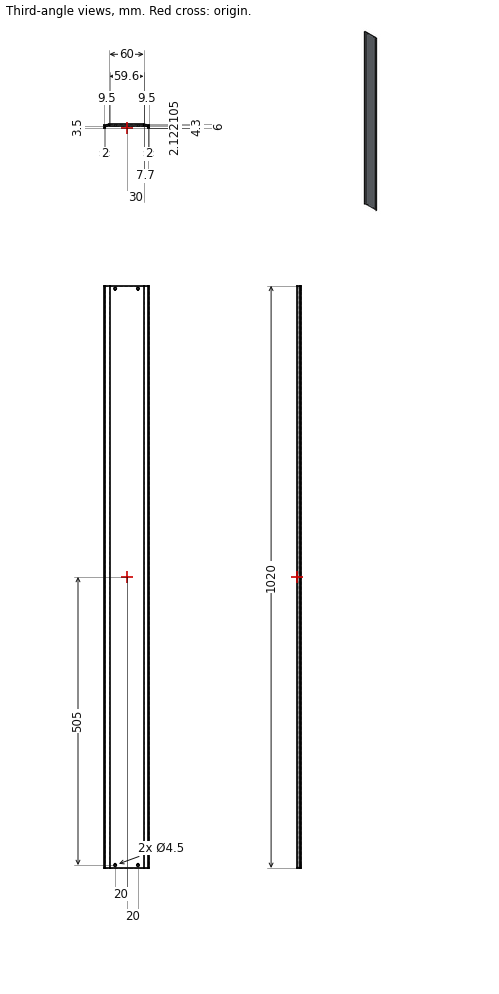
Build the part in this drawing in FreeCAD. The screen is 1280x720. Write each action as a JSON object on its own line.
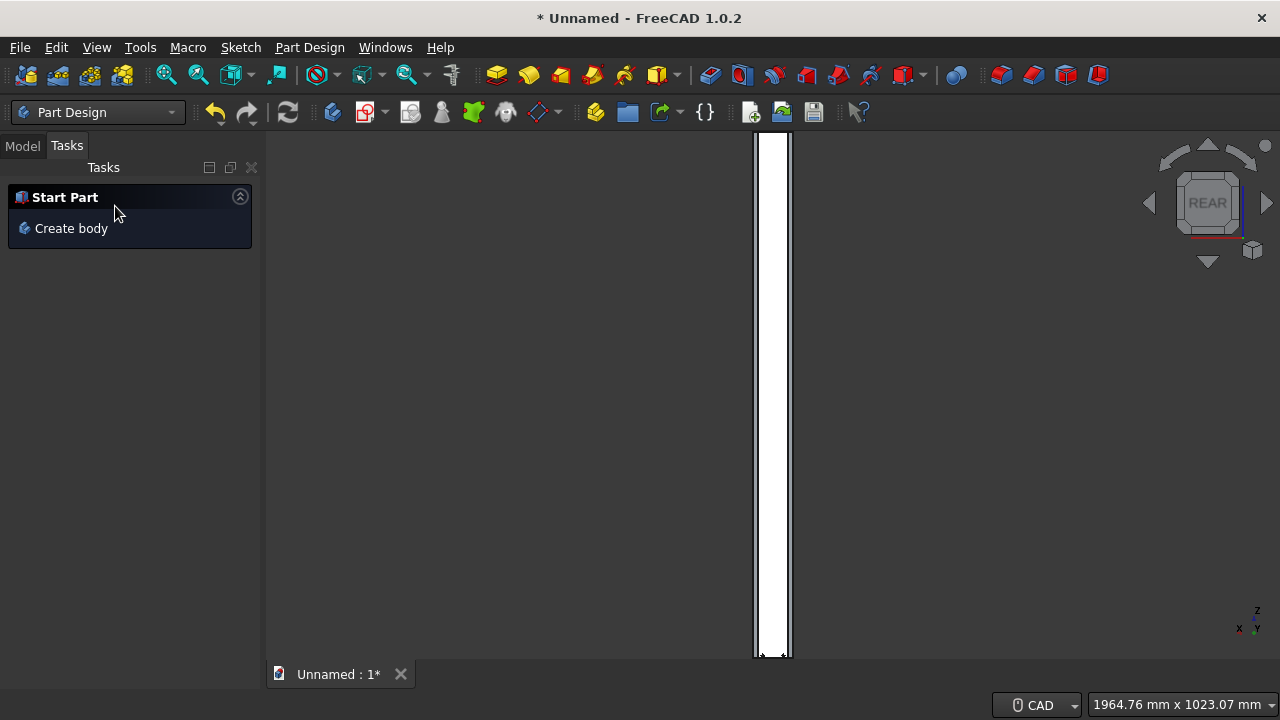
{"action": "left_click", "coordinate": [23, 145]}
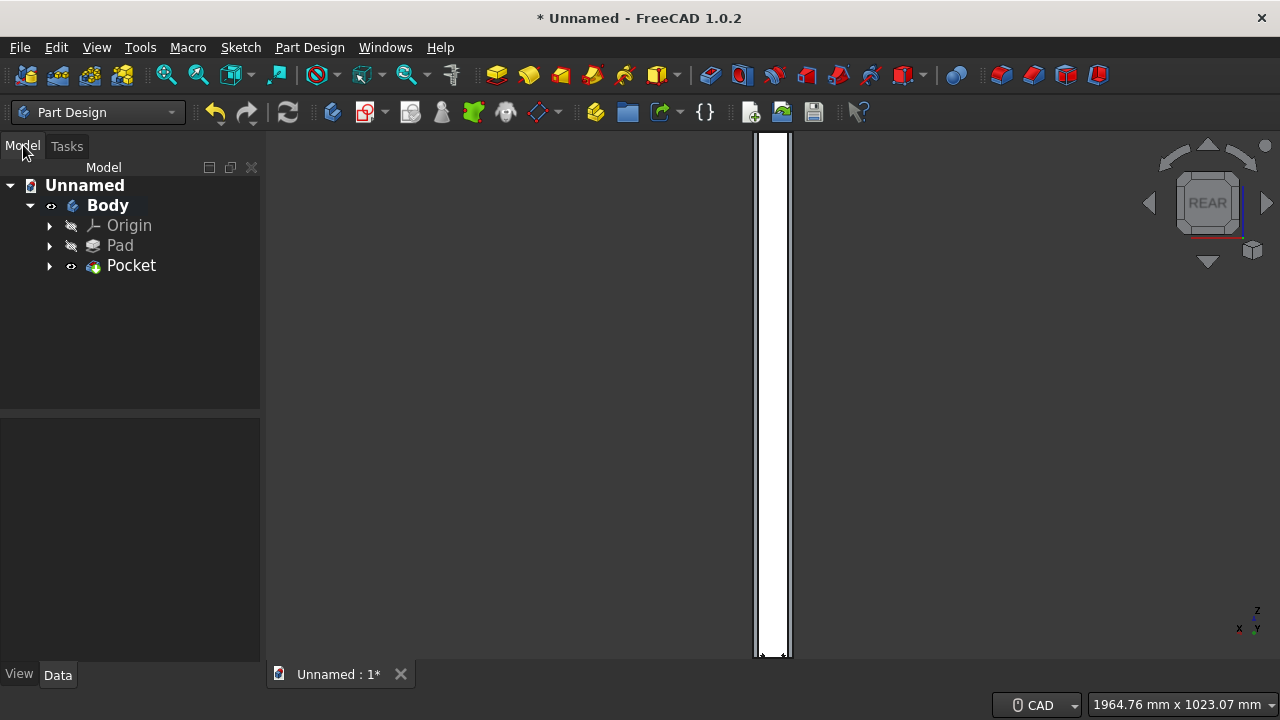
{"action": "left_click", "coordinate": [116, 266]}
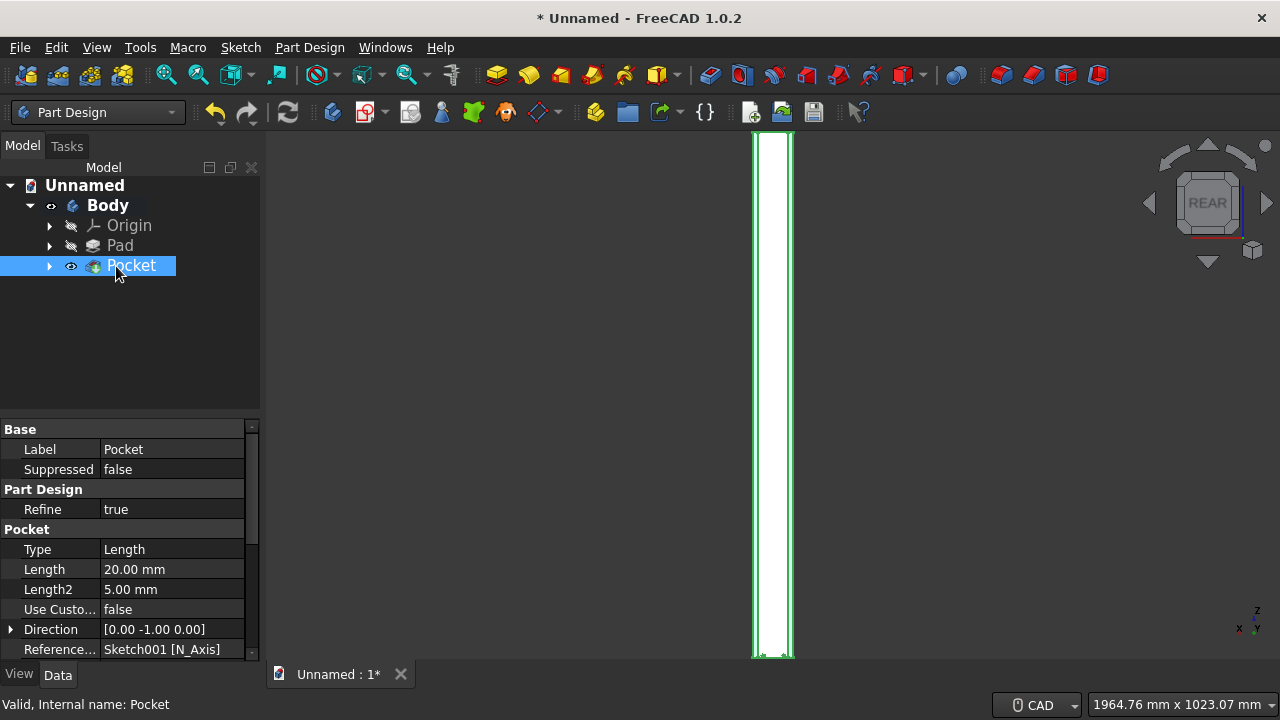
{"action": "left_click", "coordinate": [26, 76]}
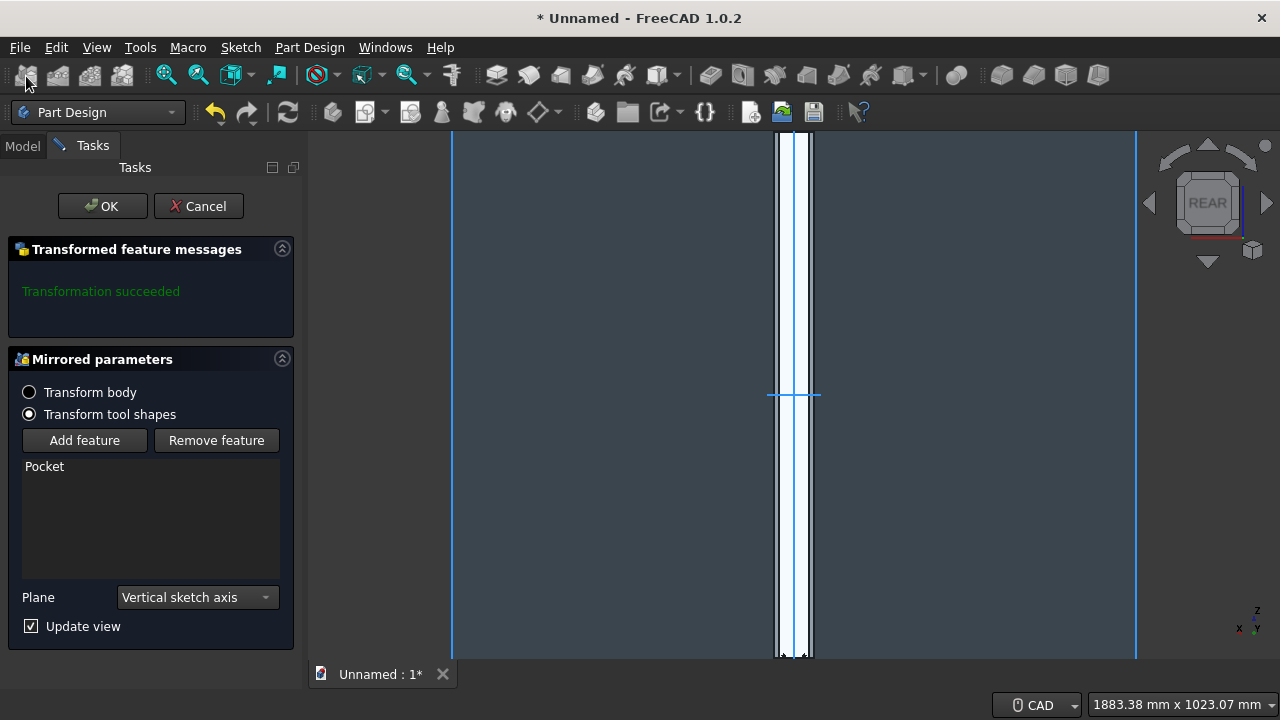
{"action": "left_click", "coordinate": [198, 598]}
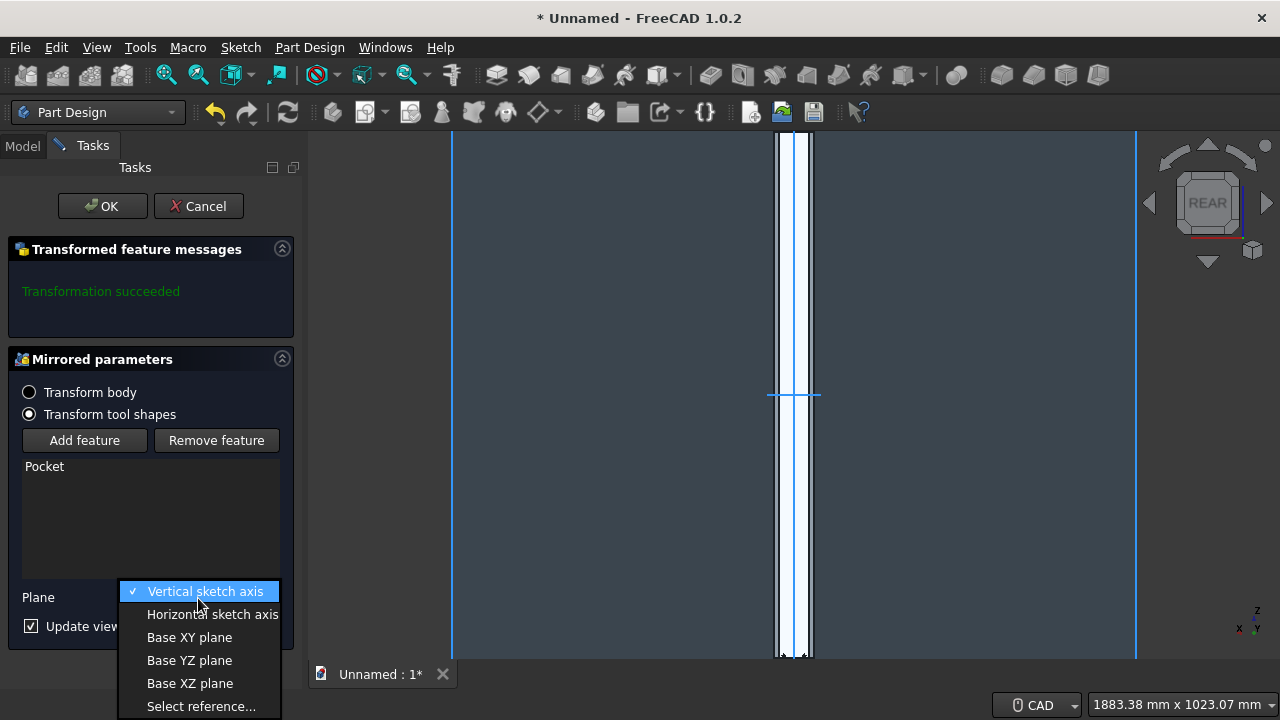
{"action": "left_click", "coordinate": [198, 638]}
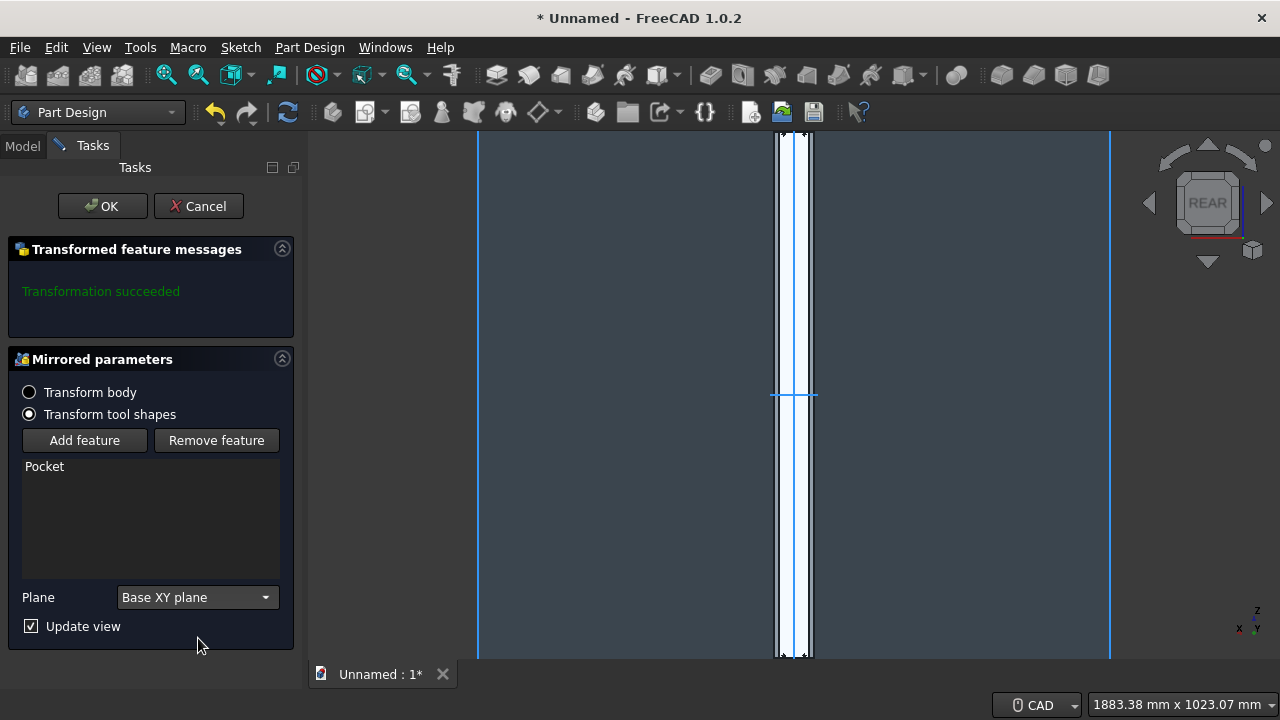
{"action": "left_click", "coordinate": [103, 206]}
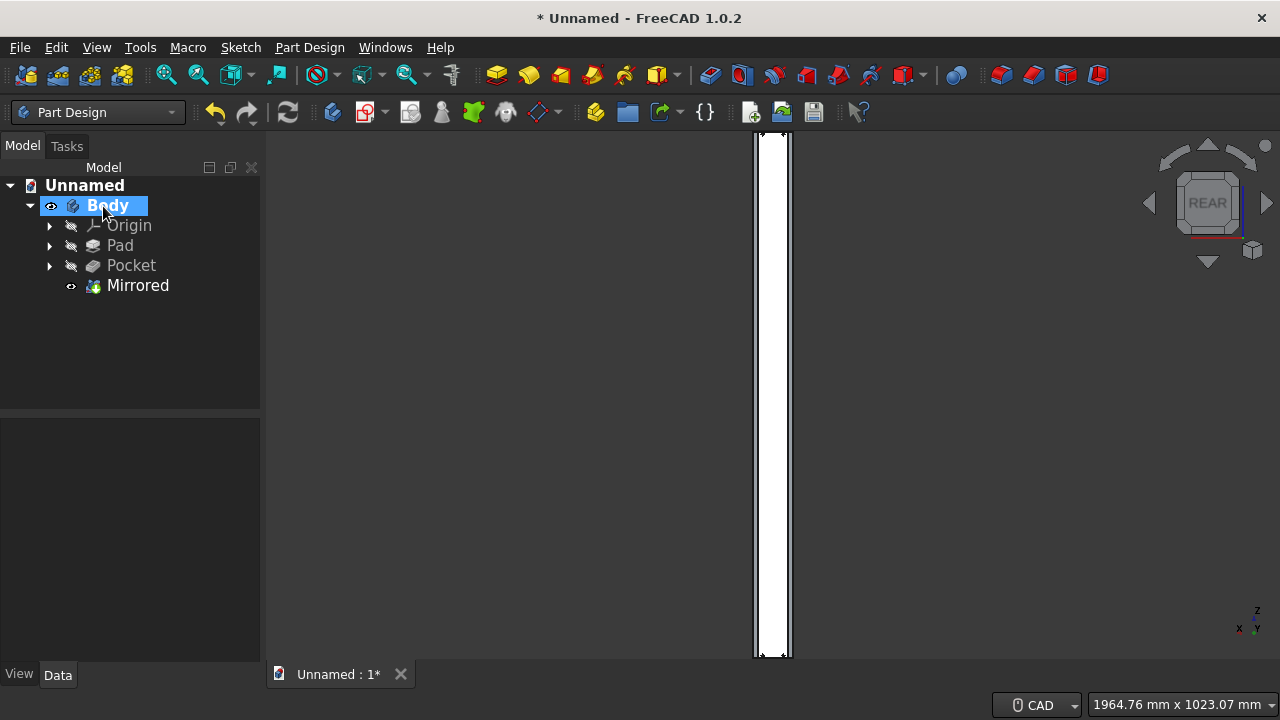
{"action": "key", "text": "0"}